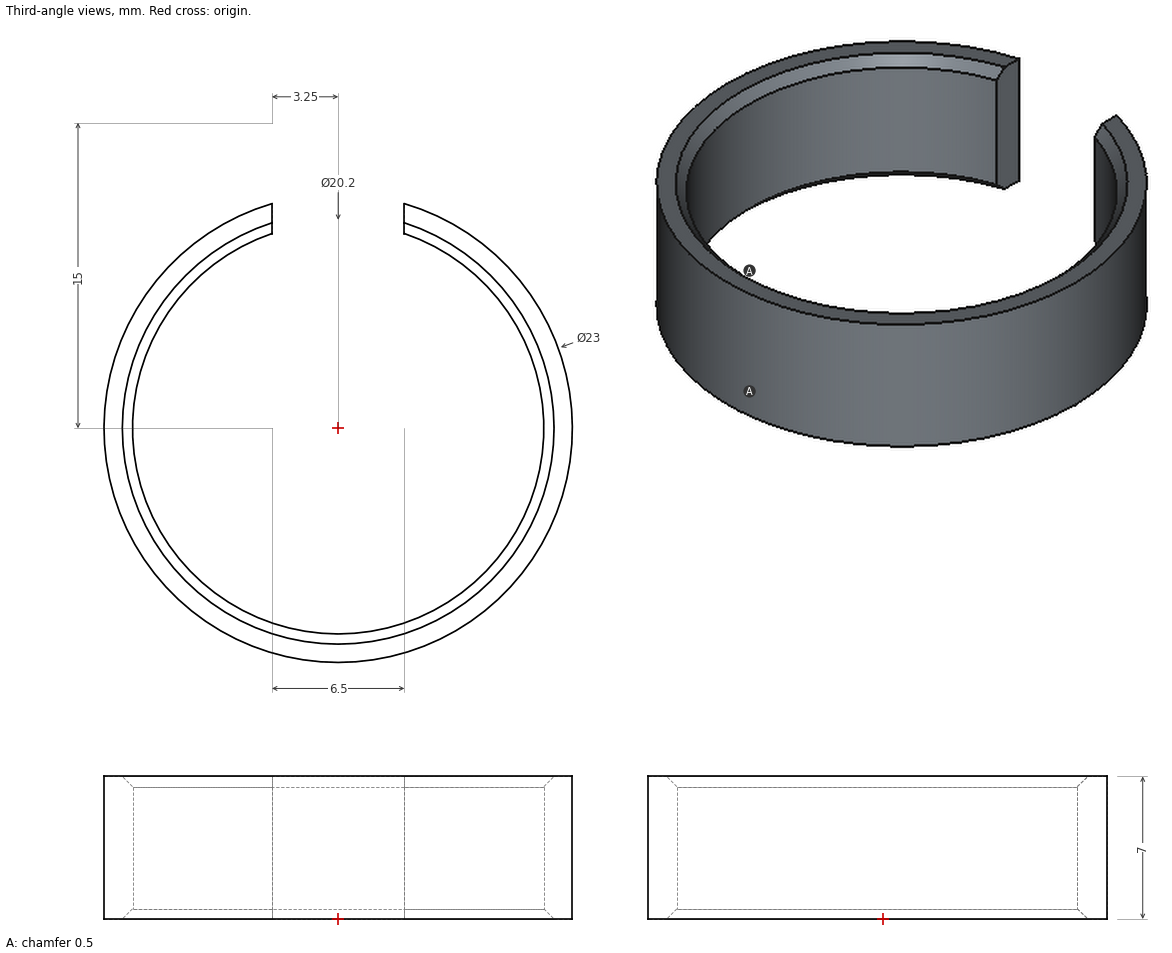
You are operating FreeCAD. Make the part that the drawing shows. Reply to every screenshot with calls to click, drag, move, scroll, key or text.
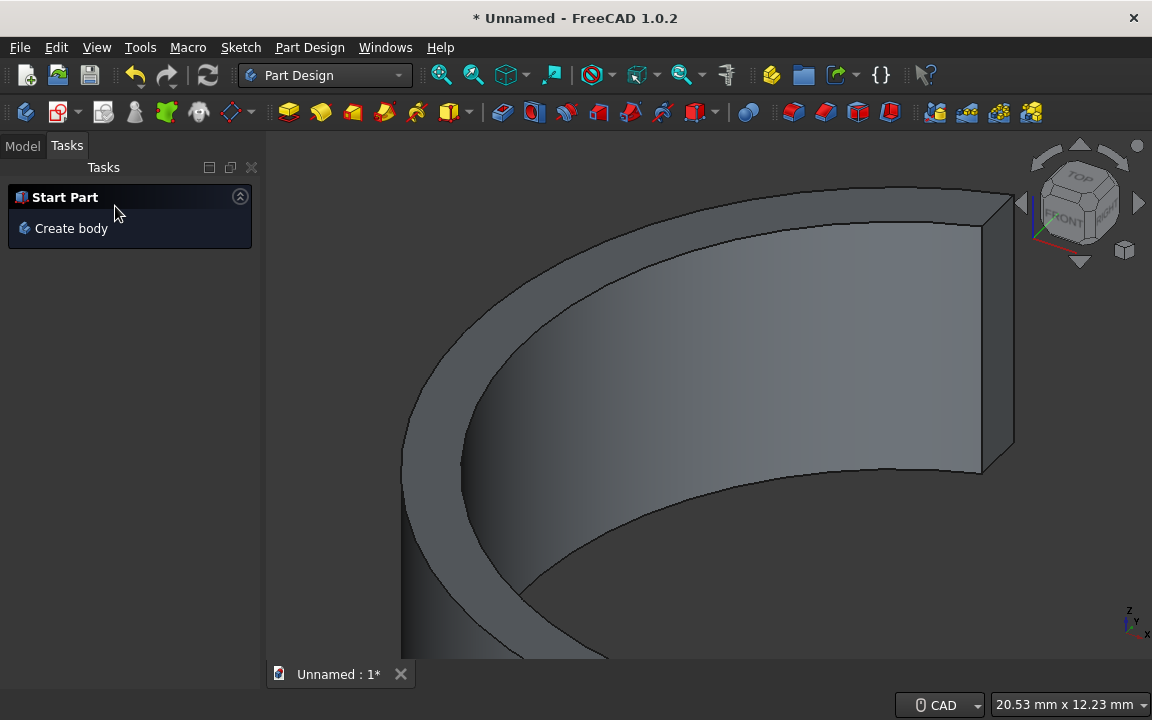
click(442, 76)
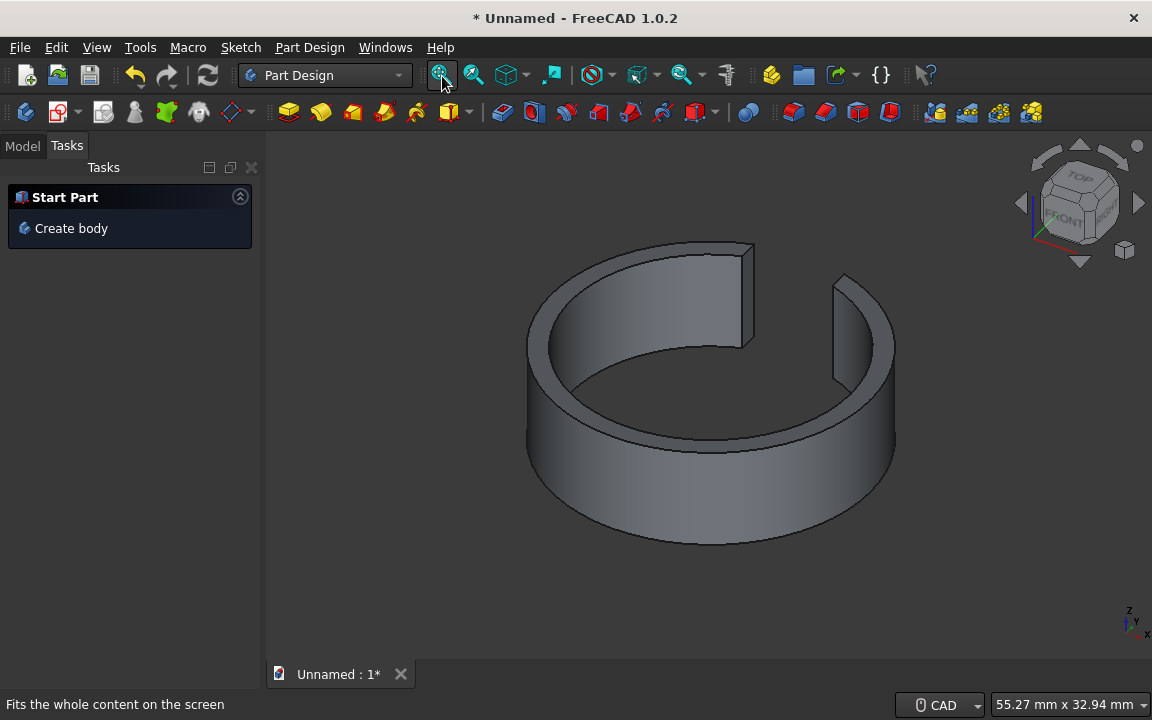
click(606, 417)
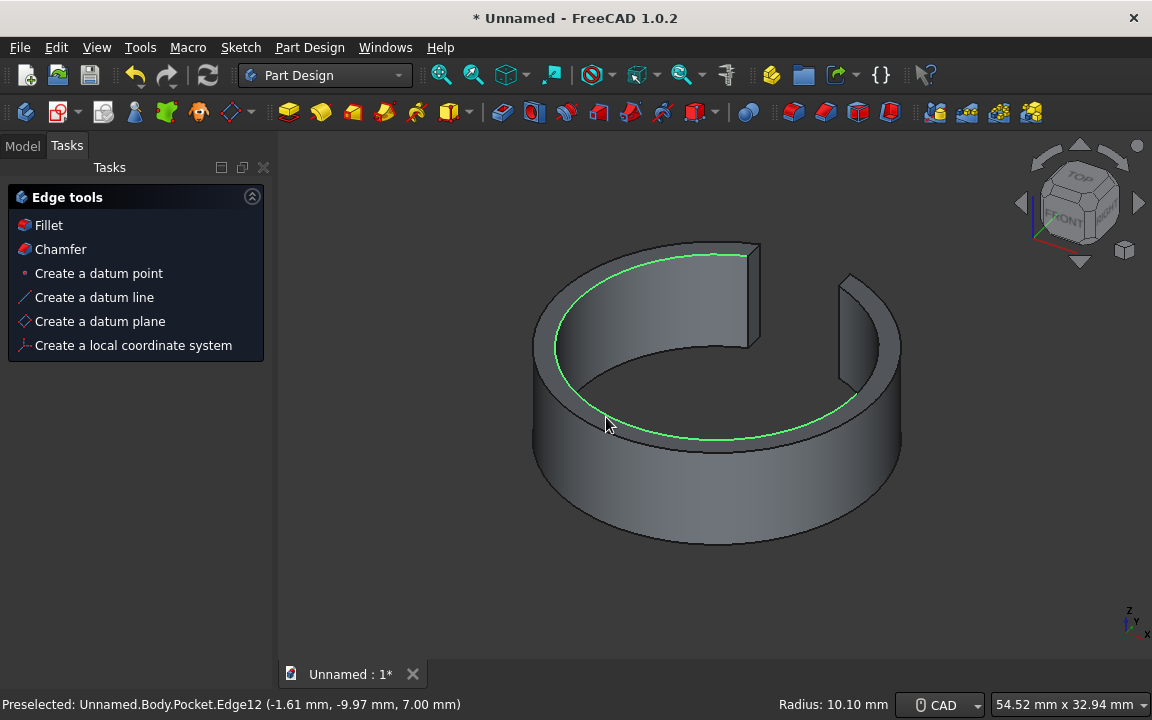
key(0)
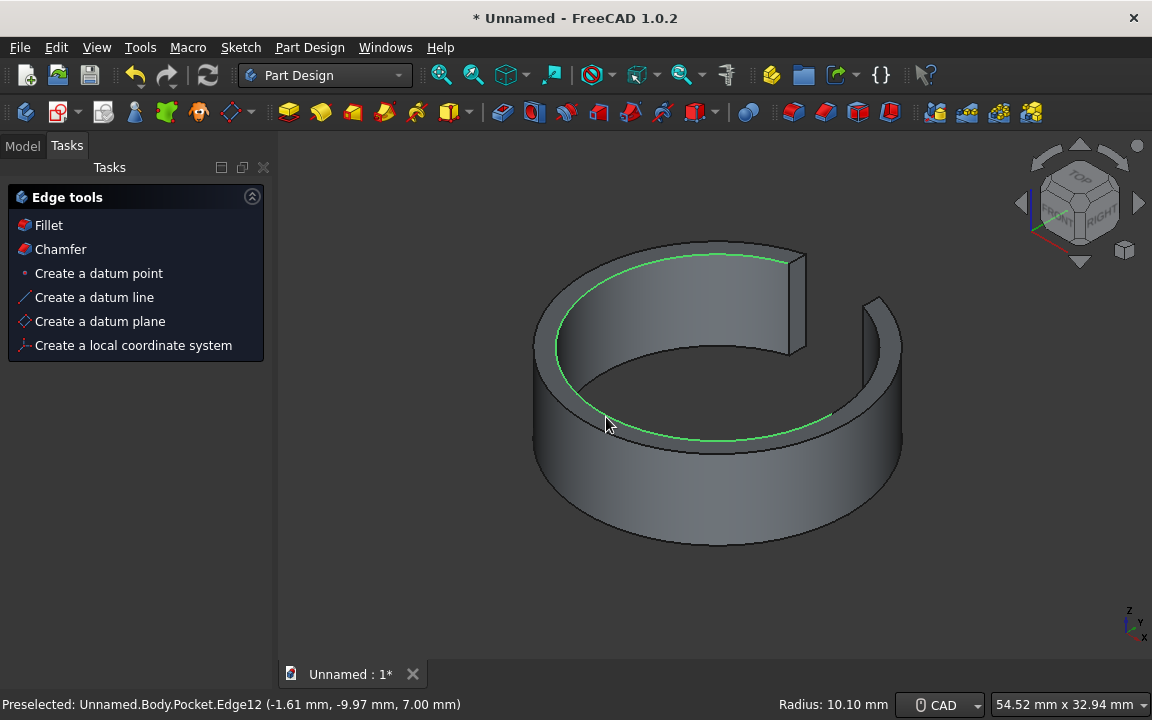
key(2)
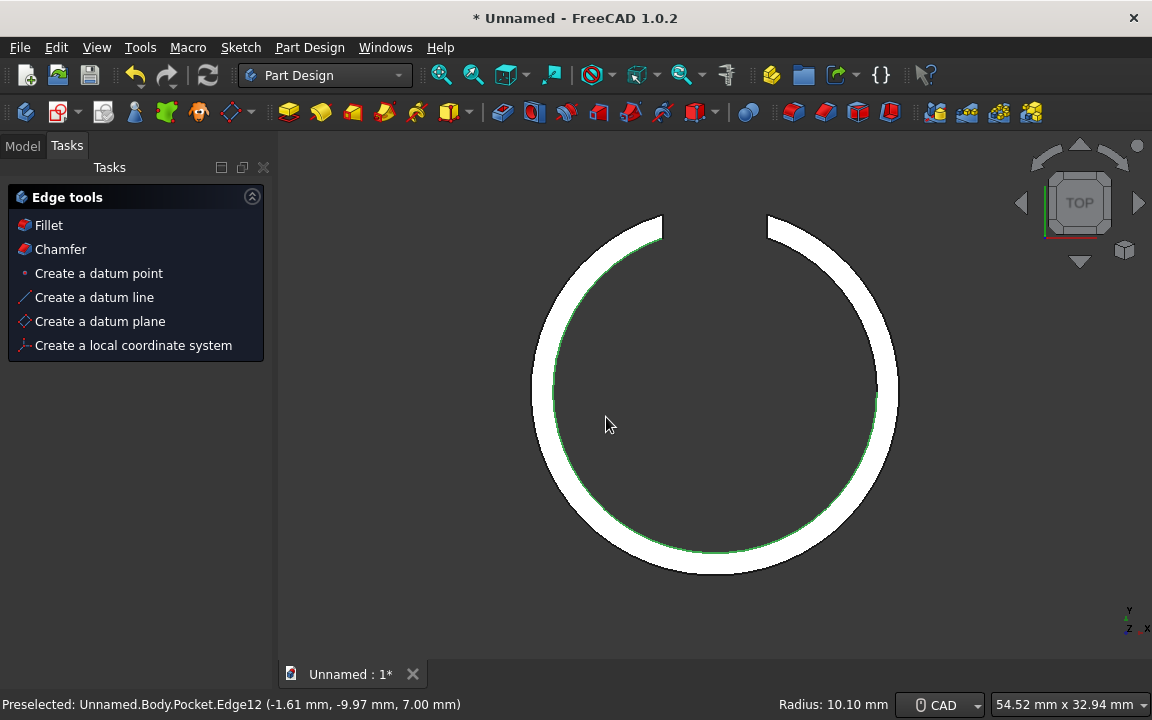
key(1)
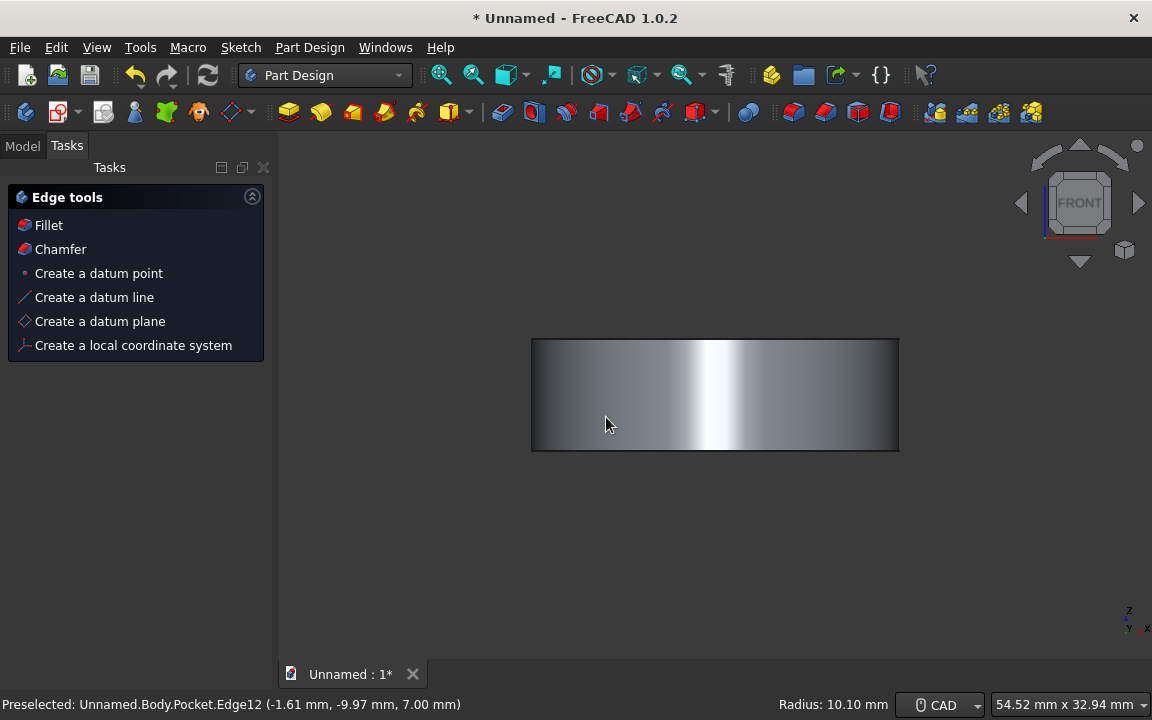
click(442, 76)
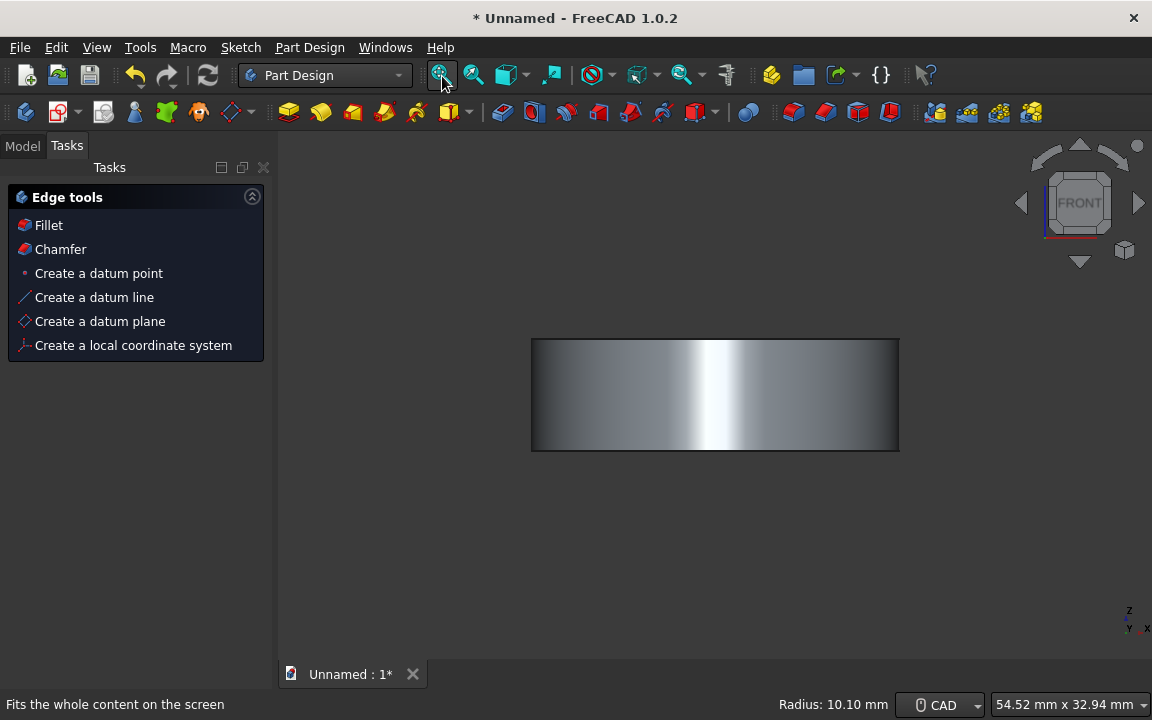
key(3)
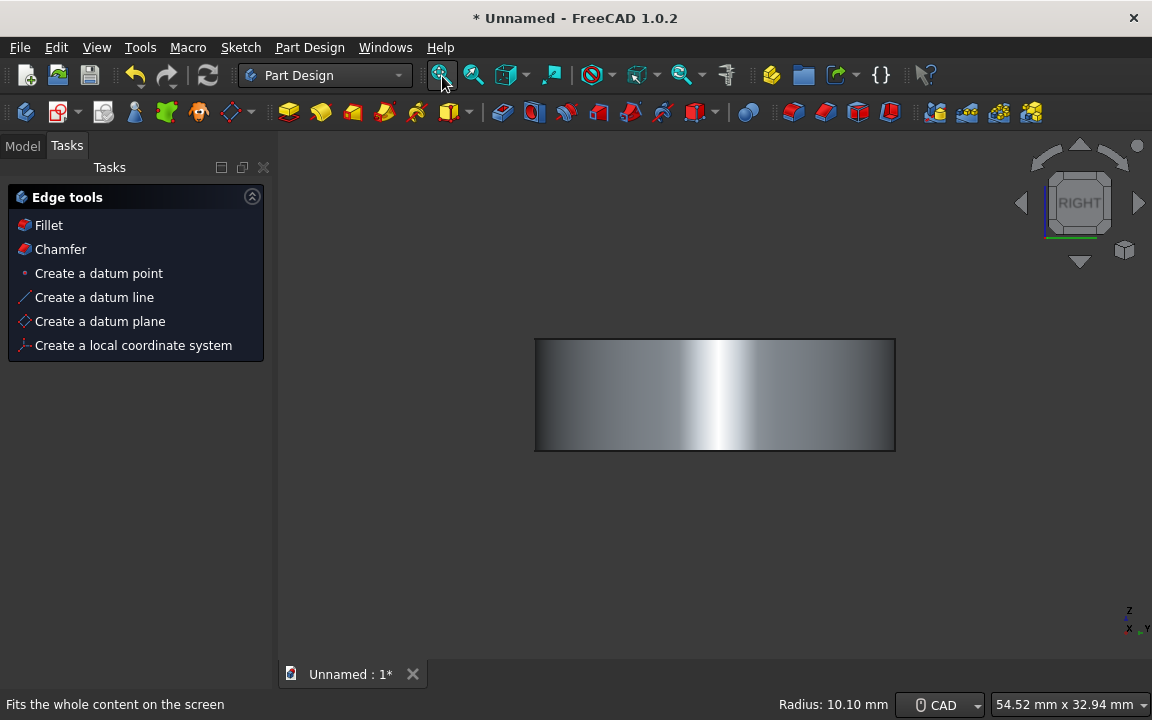
click(442, 76)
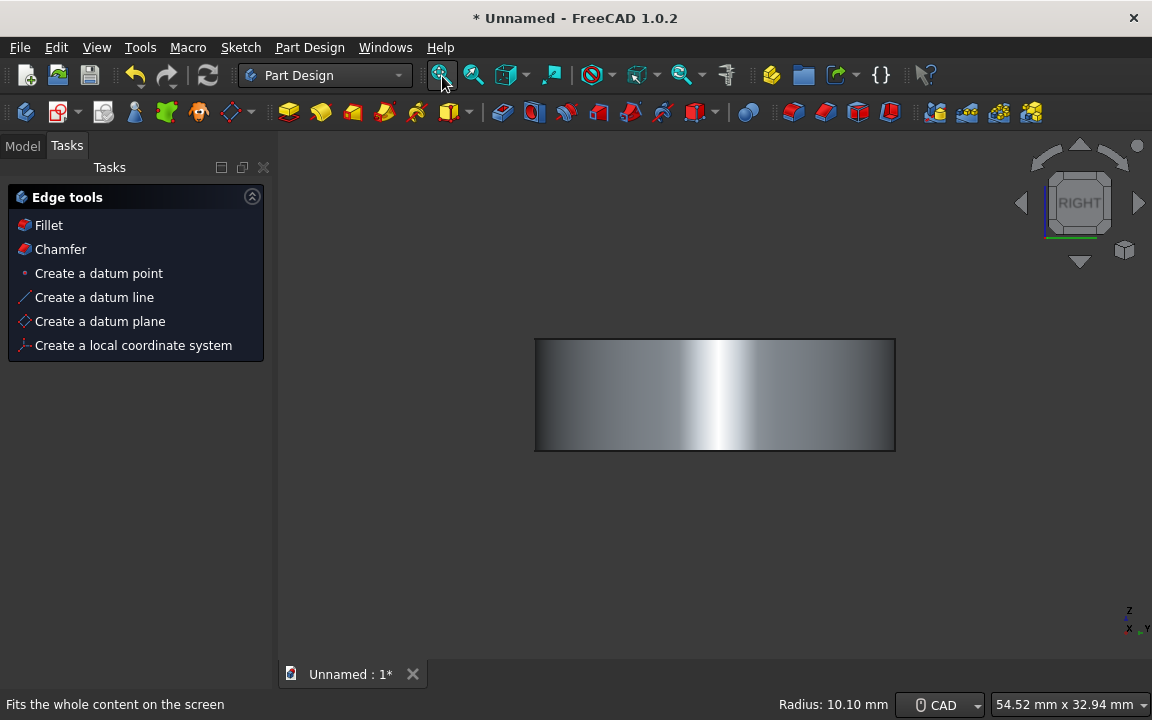
key(5)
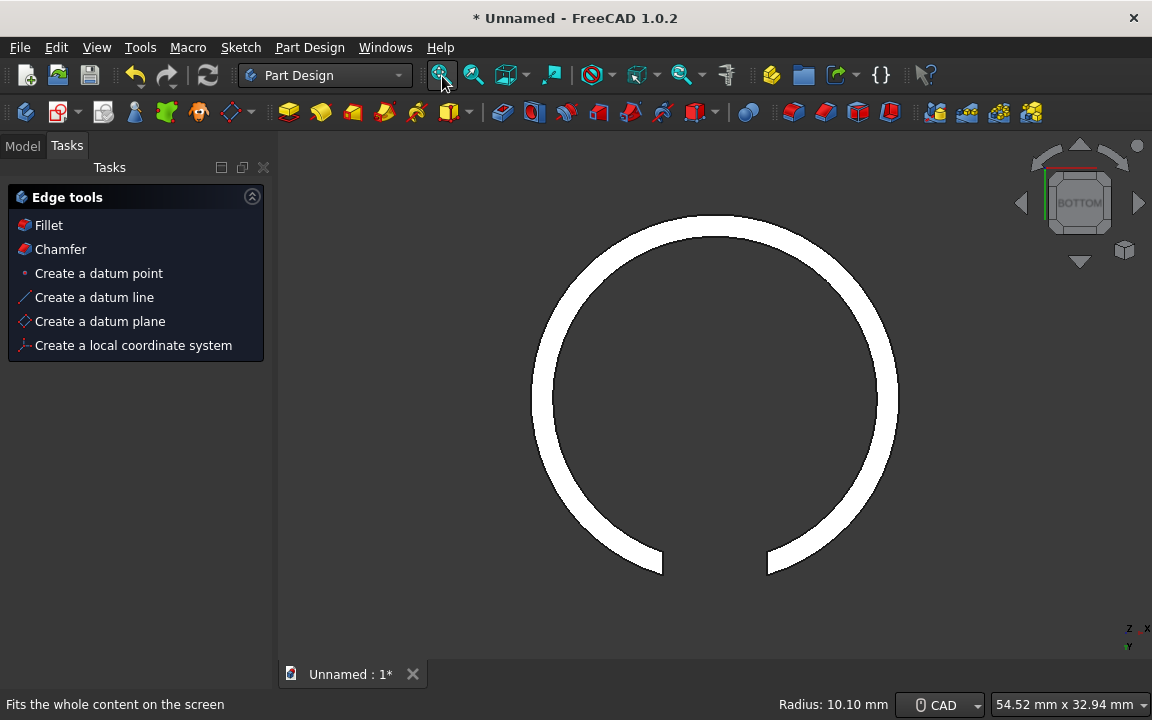
click(621, 266, ctrl)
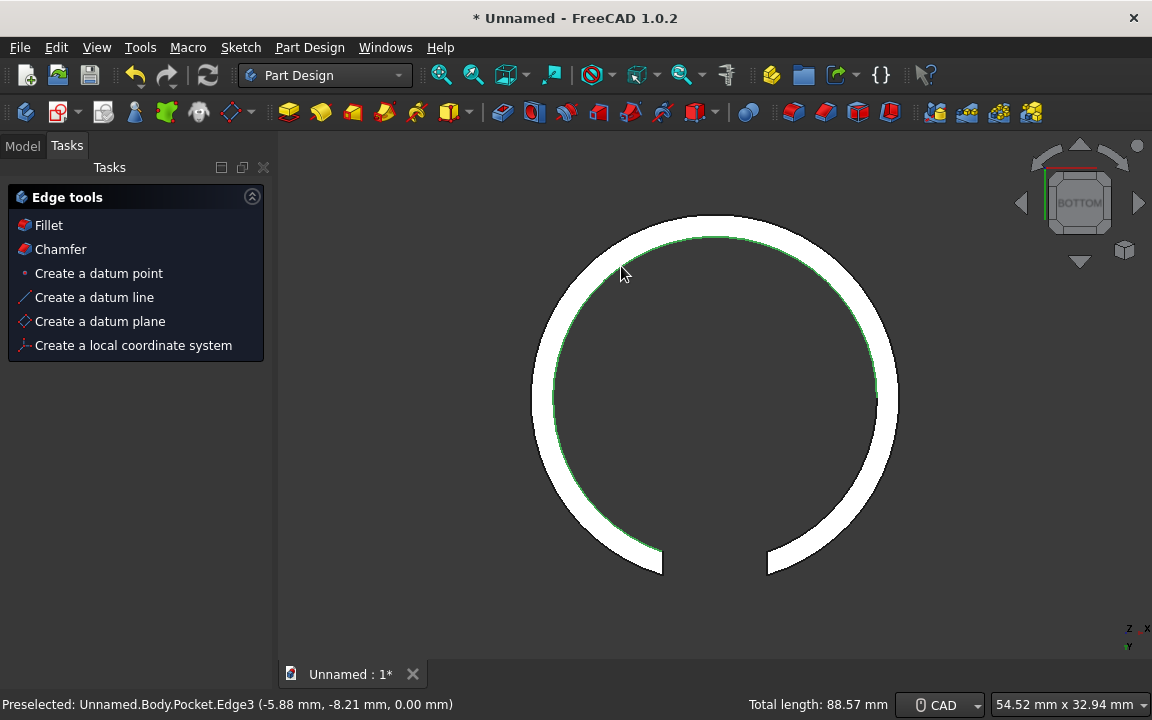
click(826, 112)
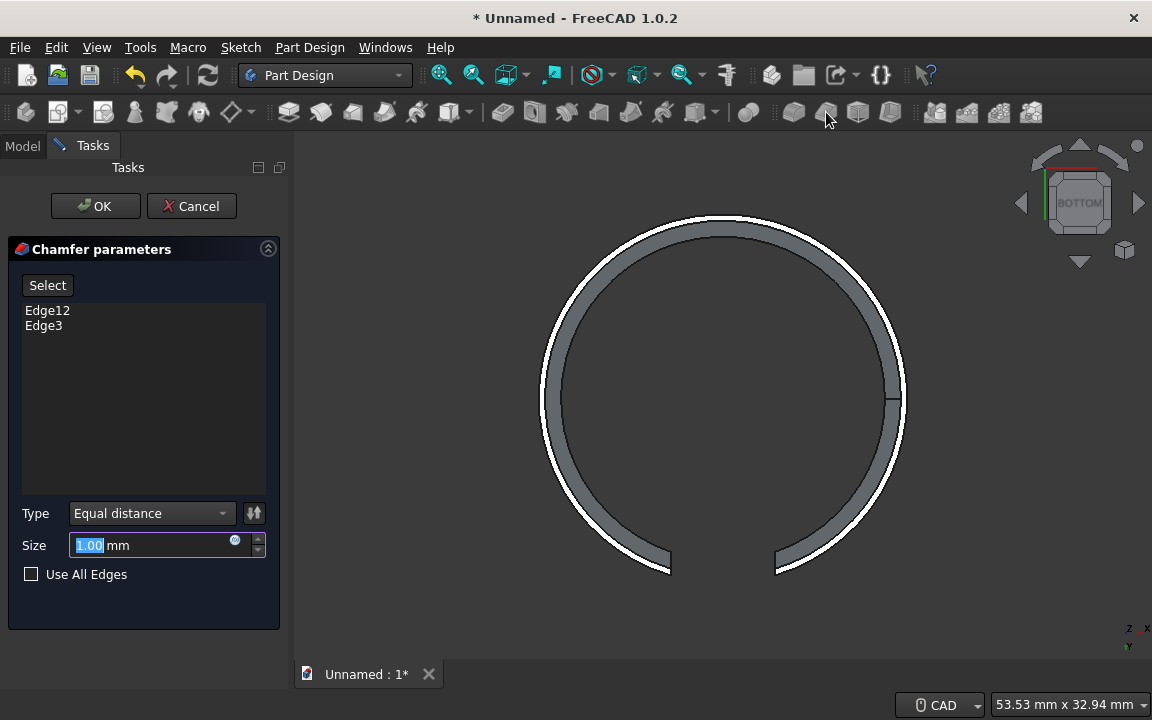
text(0.5)
key(Tab)